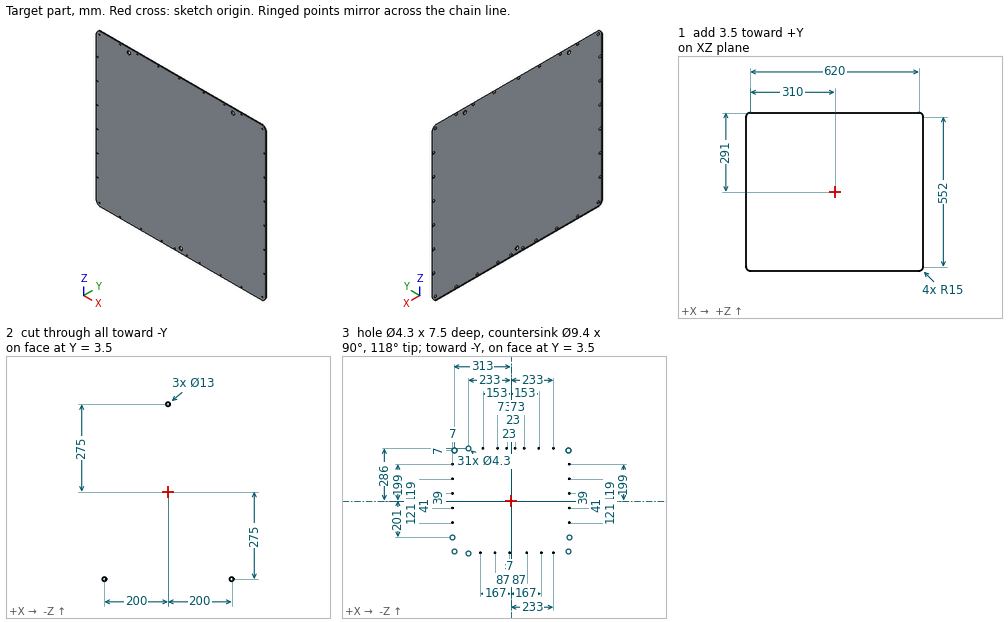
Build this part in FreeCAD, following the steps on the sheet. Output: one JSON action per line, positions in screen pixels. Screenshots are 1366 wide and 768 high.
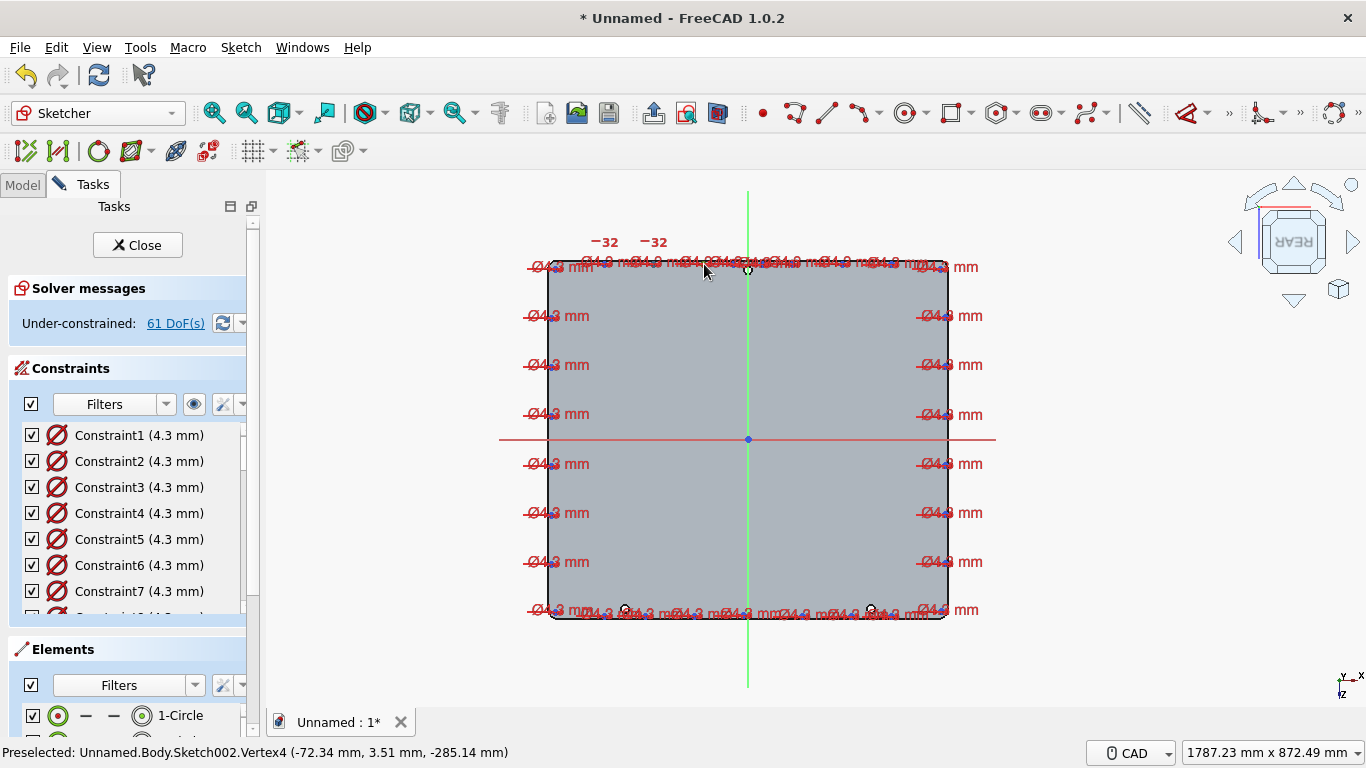
{"action": "key", "text": "h"}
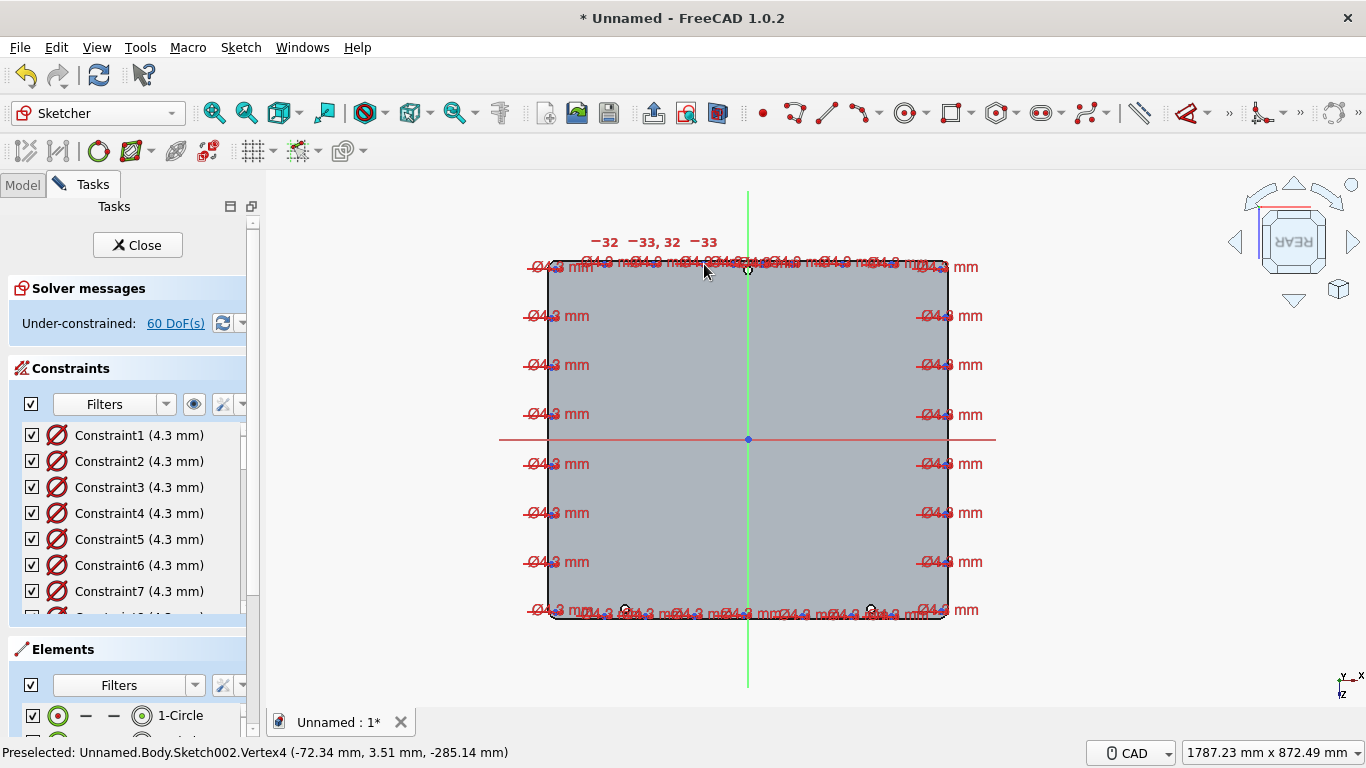
{"action": "left_click", "coordinate": [704, 264]}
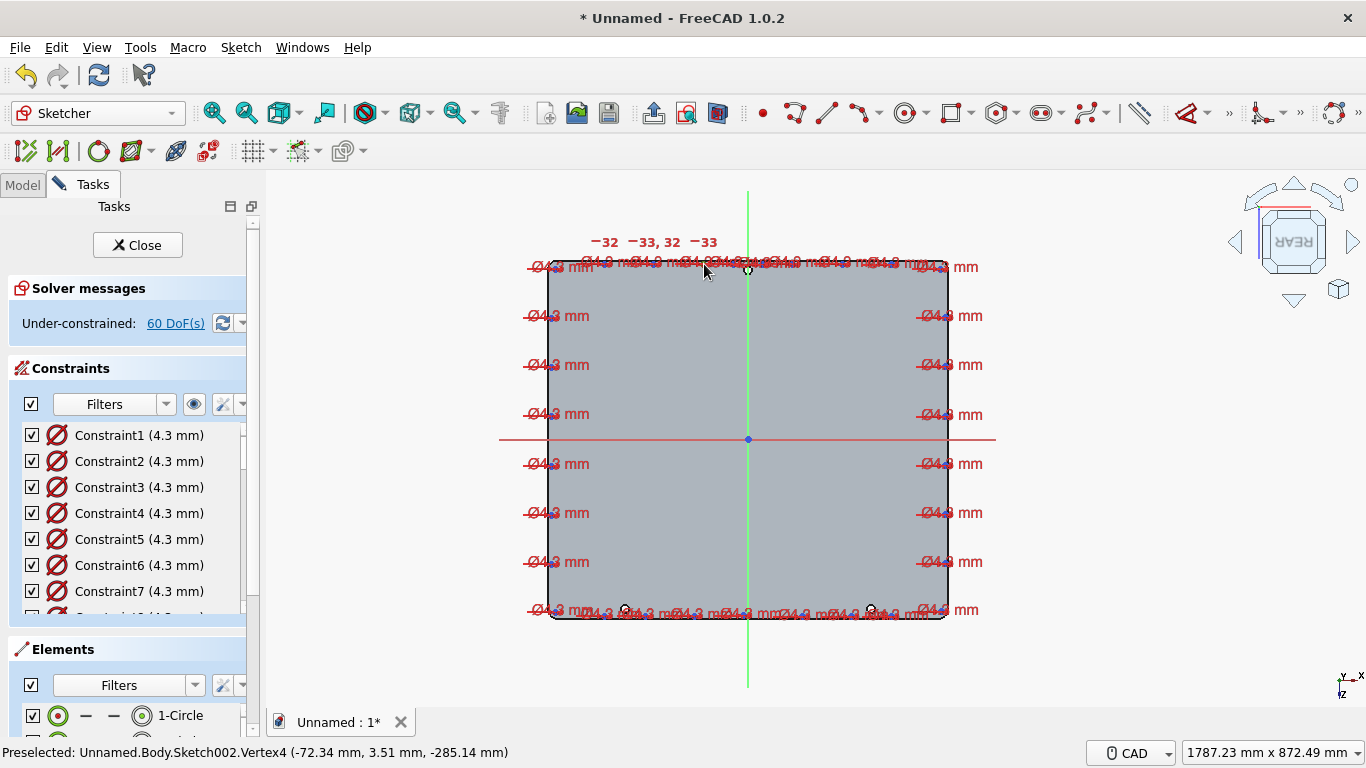
{"action": "left_click", "coordinate": [734, 264]}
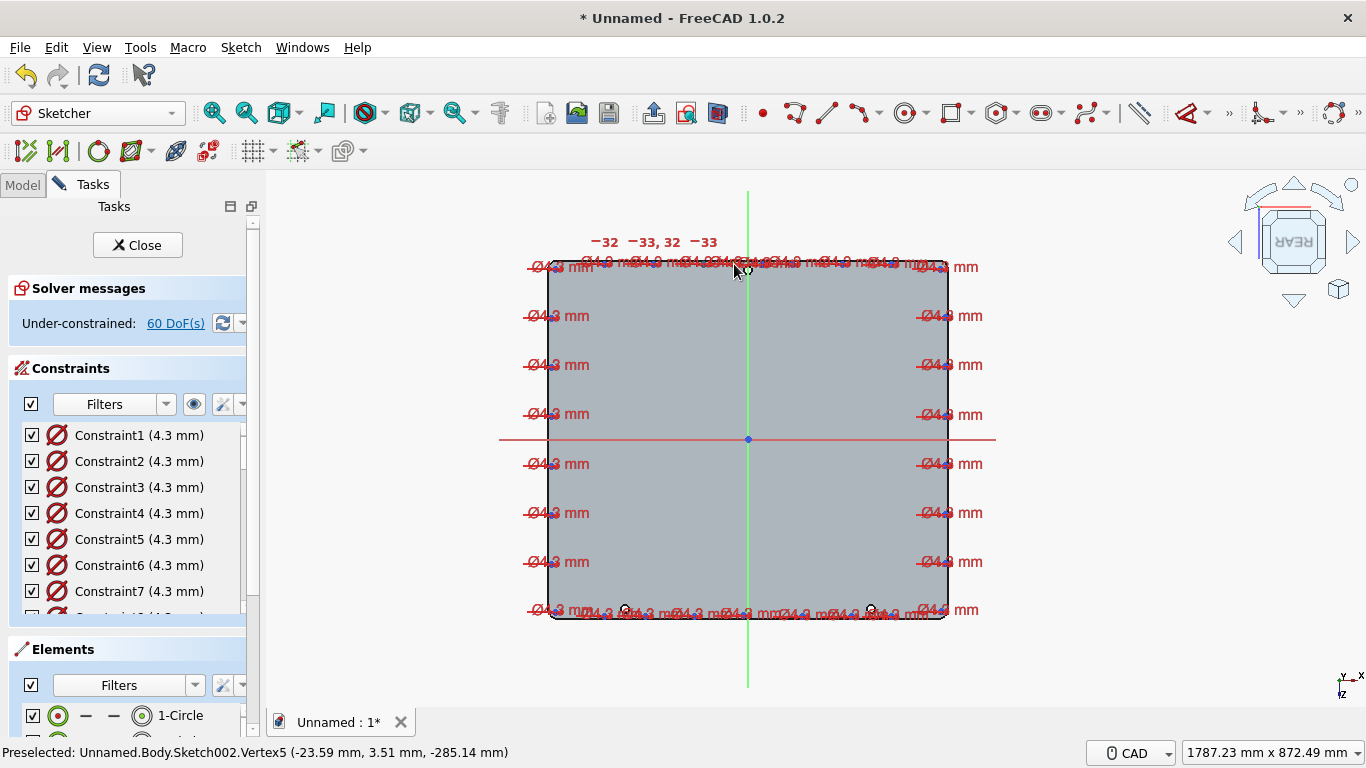
{"action": "key", "text": "h"}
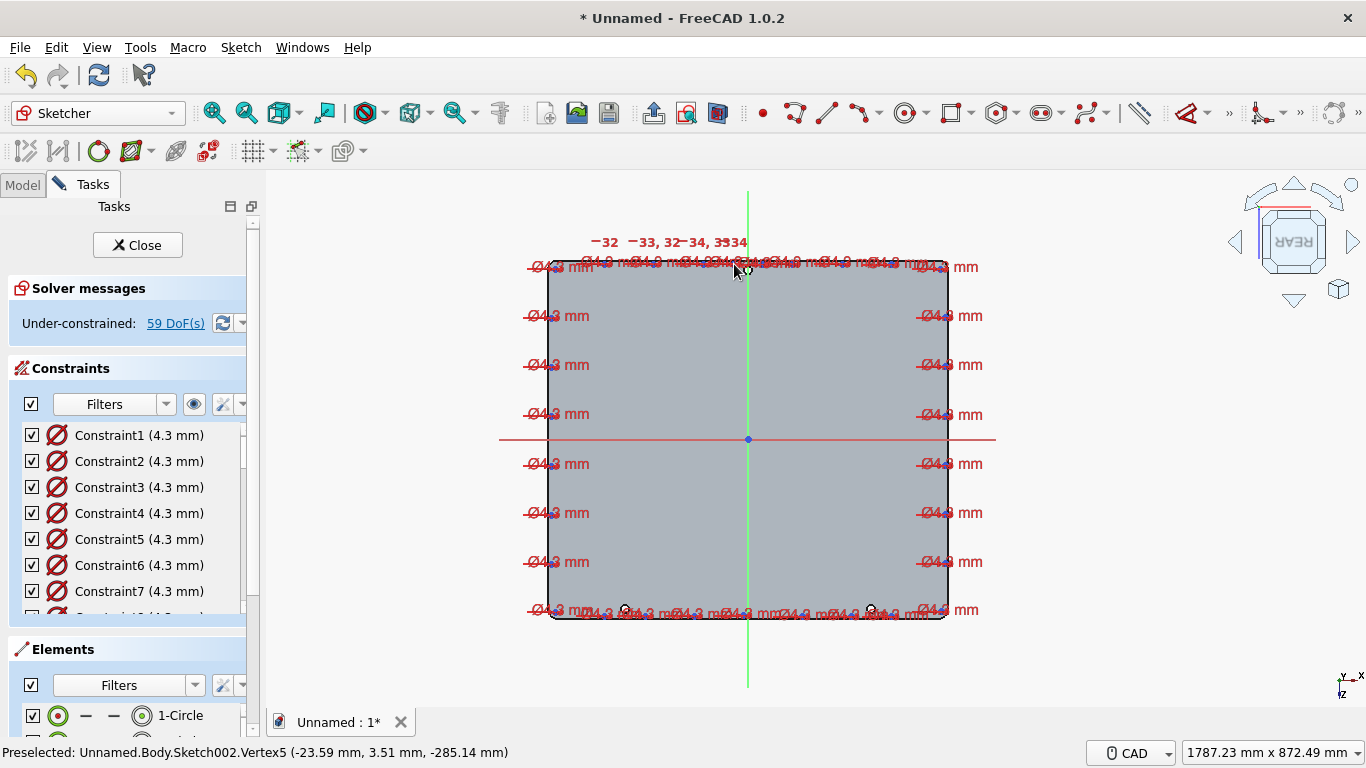
{"action": "left_click", "coordinate": [734, 264]}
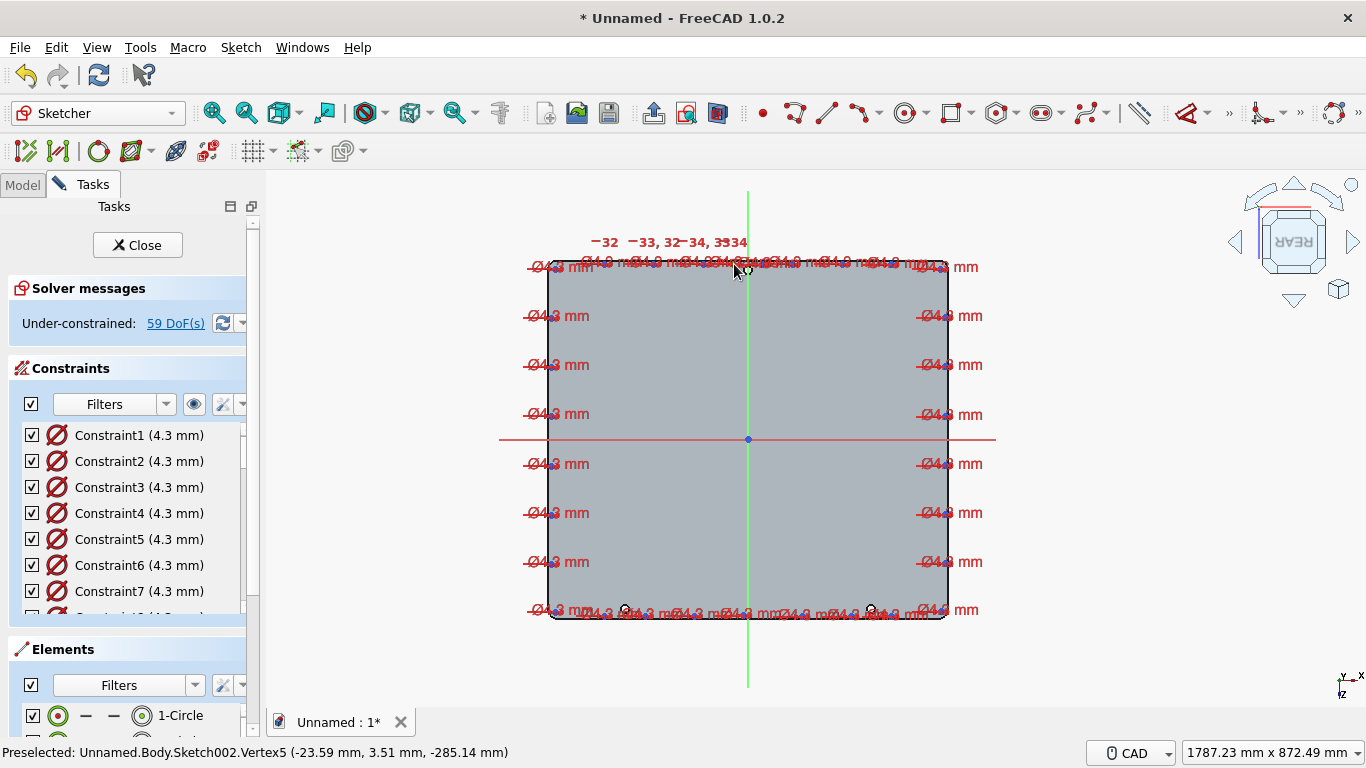
{"action": "left_click", "coordinate": [793, 264]}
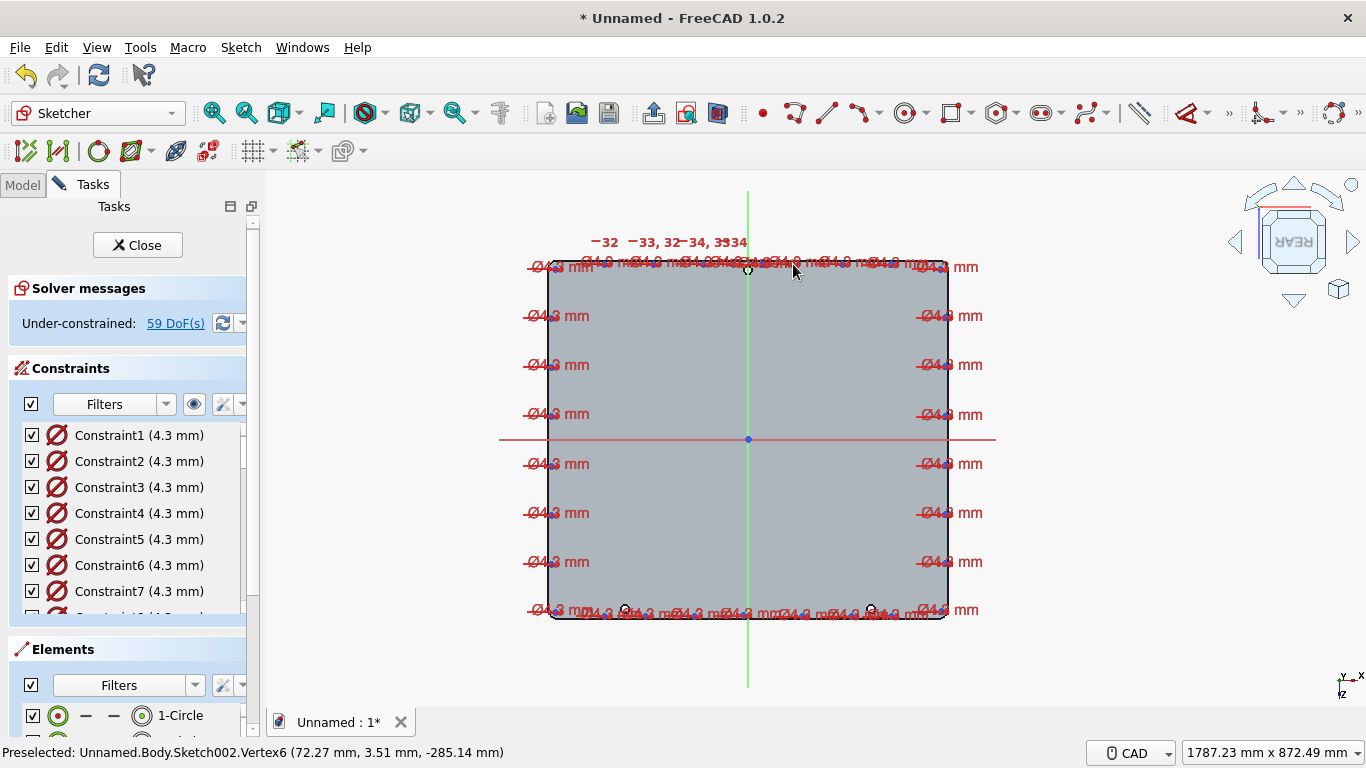
{"action": "key", "text": "h"}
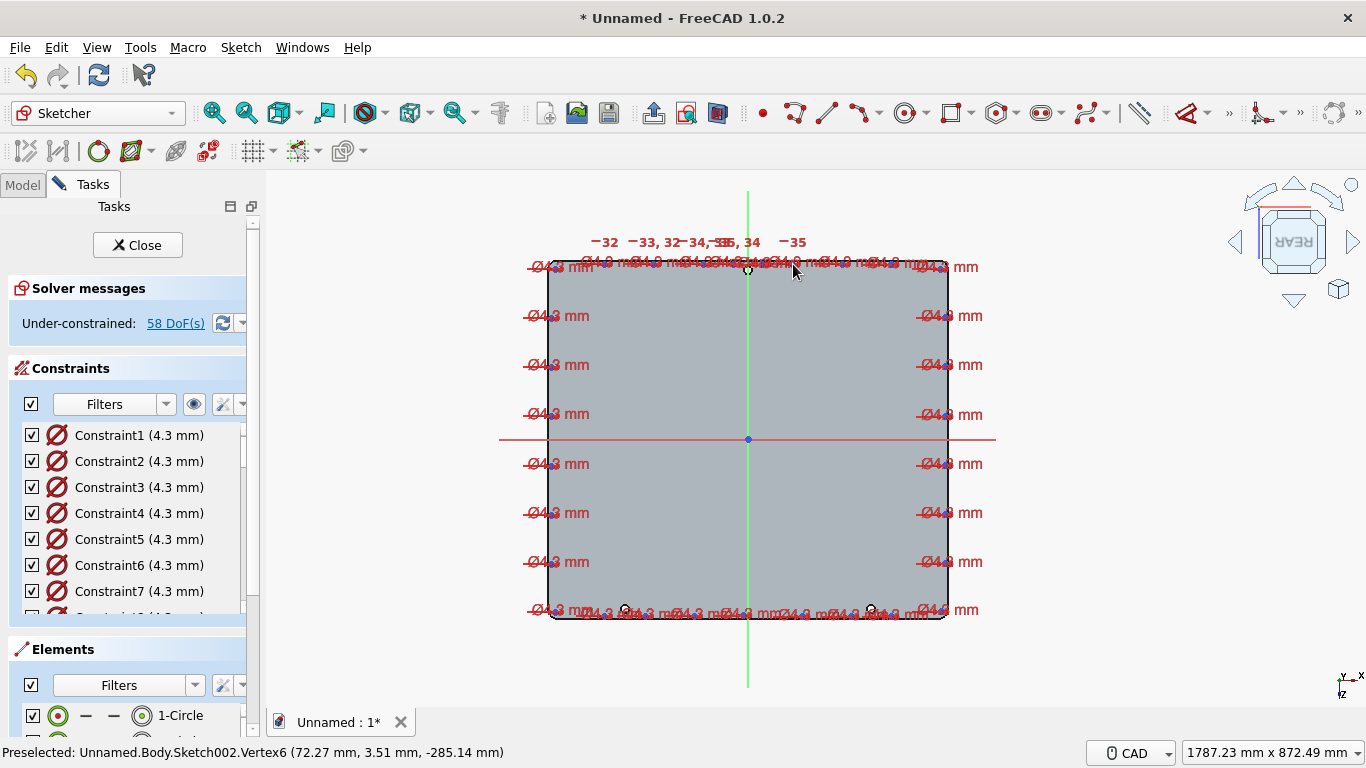
{"action": "left_click", "coordinate": [793, 264]}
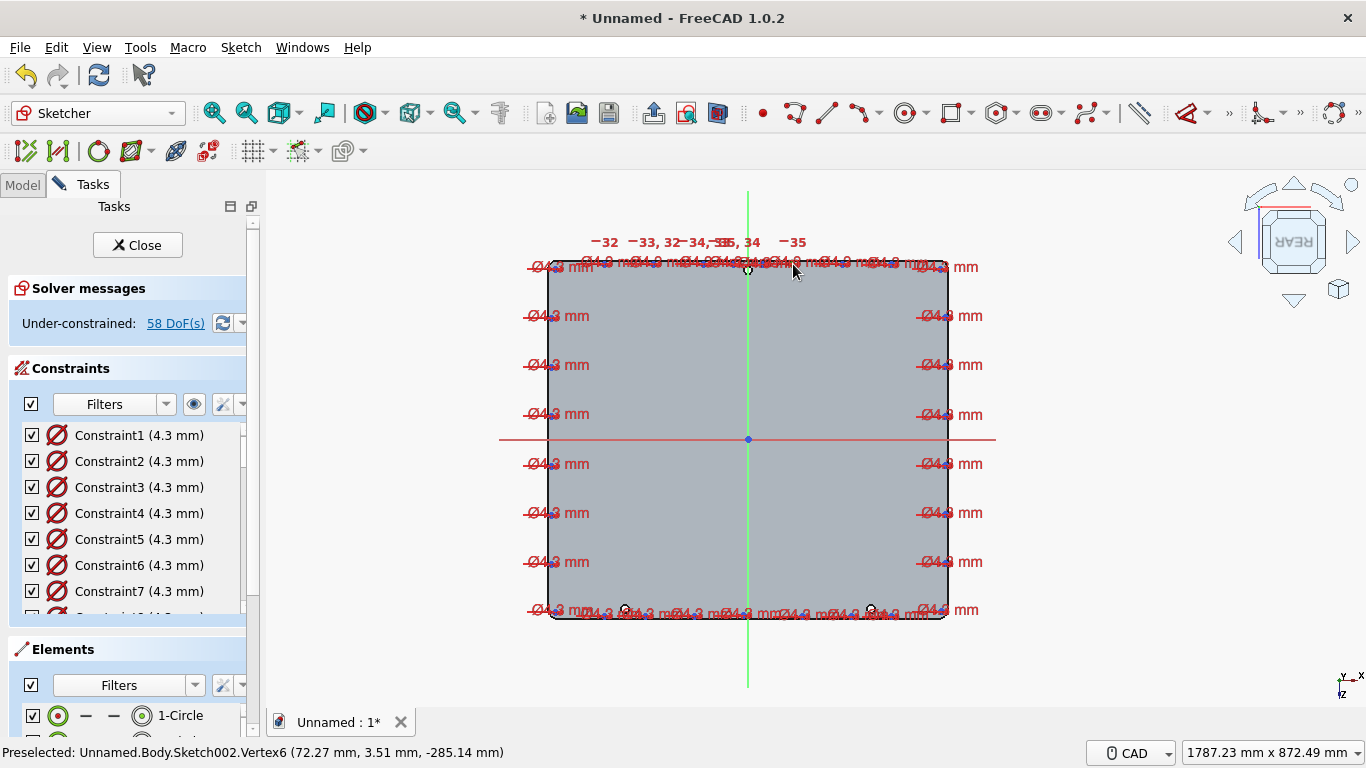
{"action": "left_click", "coordinate": [843, 264]}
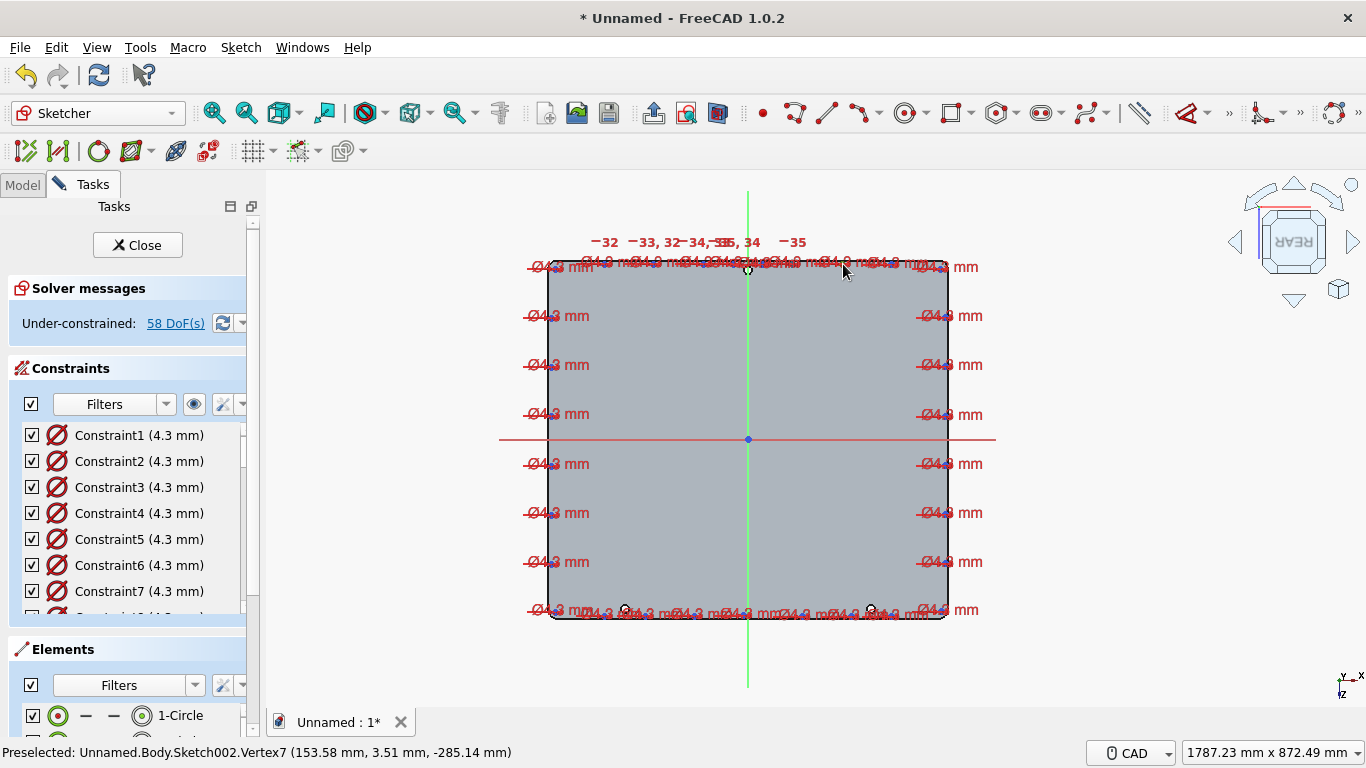
{"action": "key", "text": "h"}